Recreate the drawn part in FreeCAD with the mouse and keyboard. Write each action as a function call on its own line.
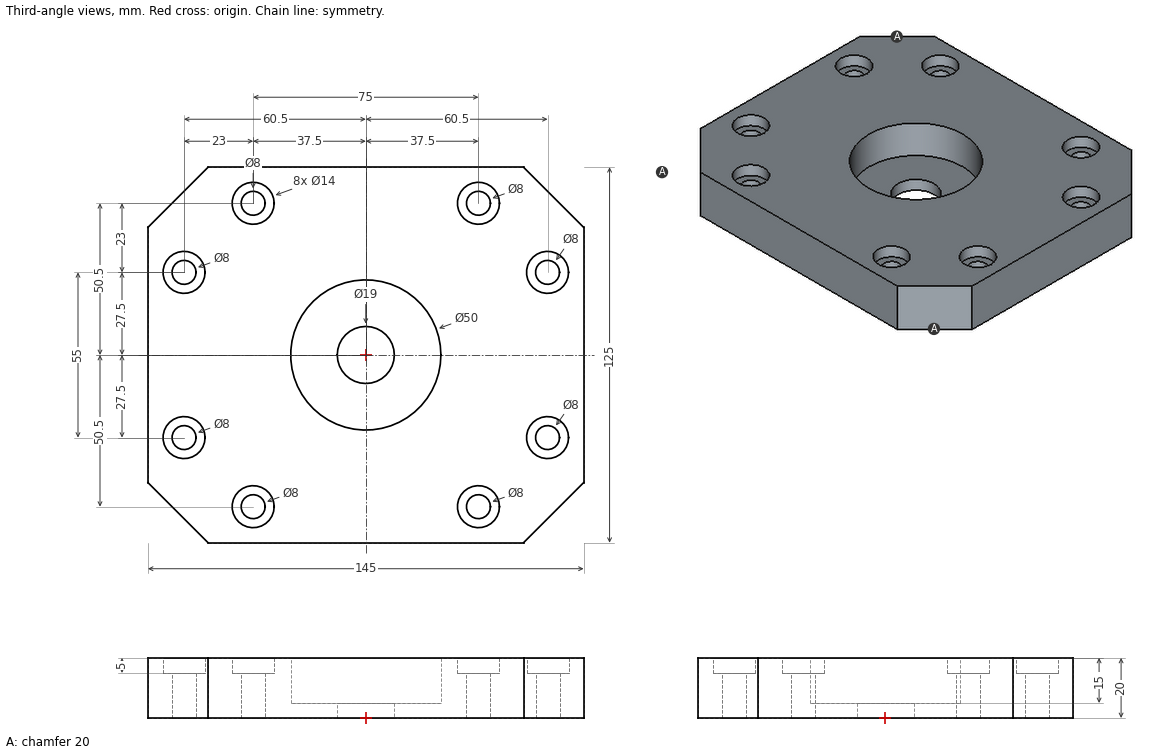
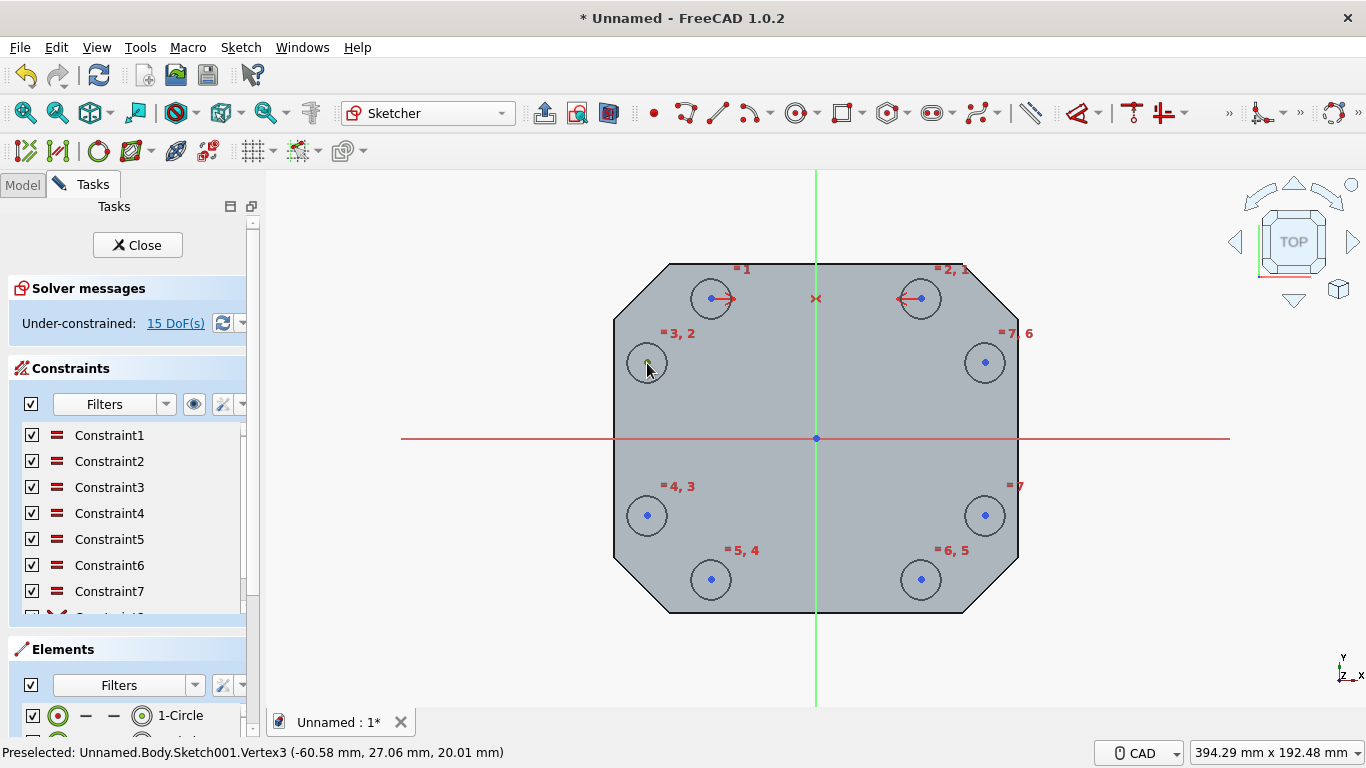
click(647, 516)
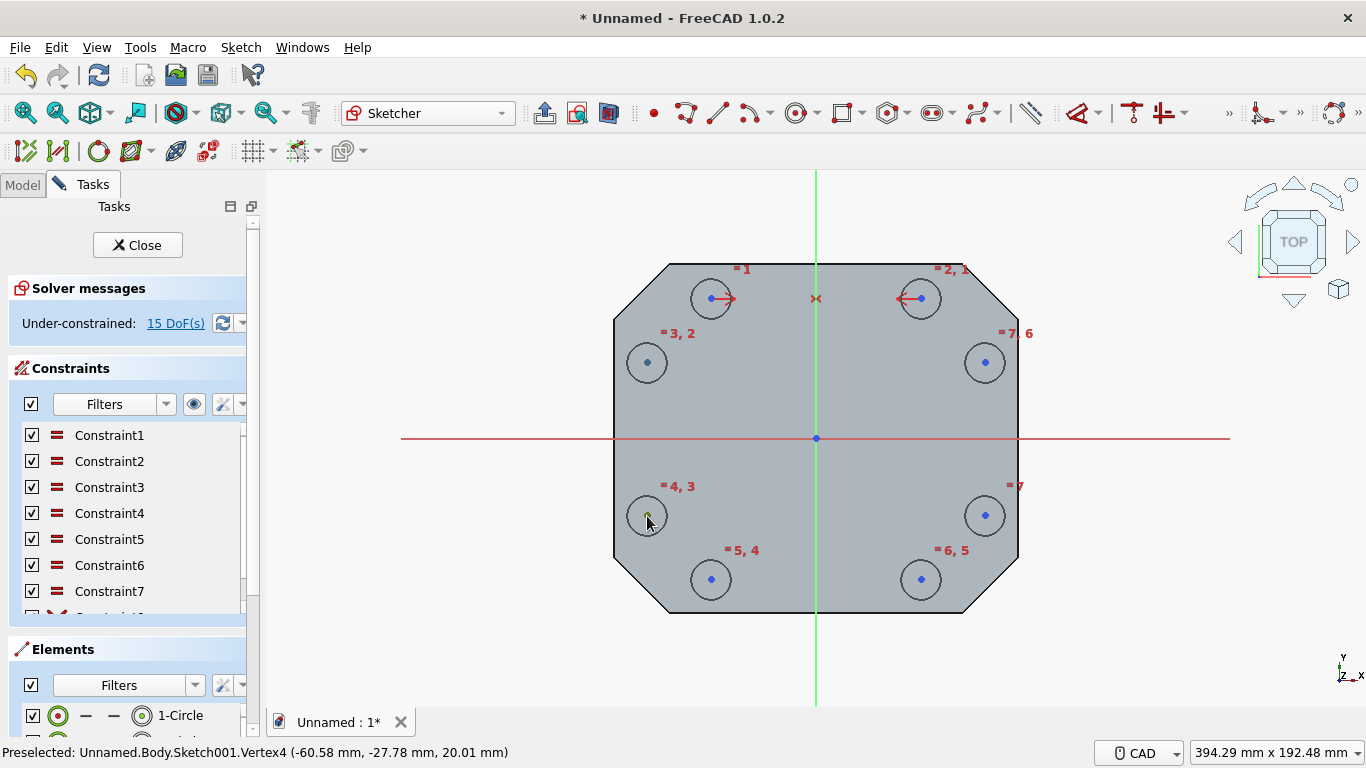
click(424, 438)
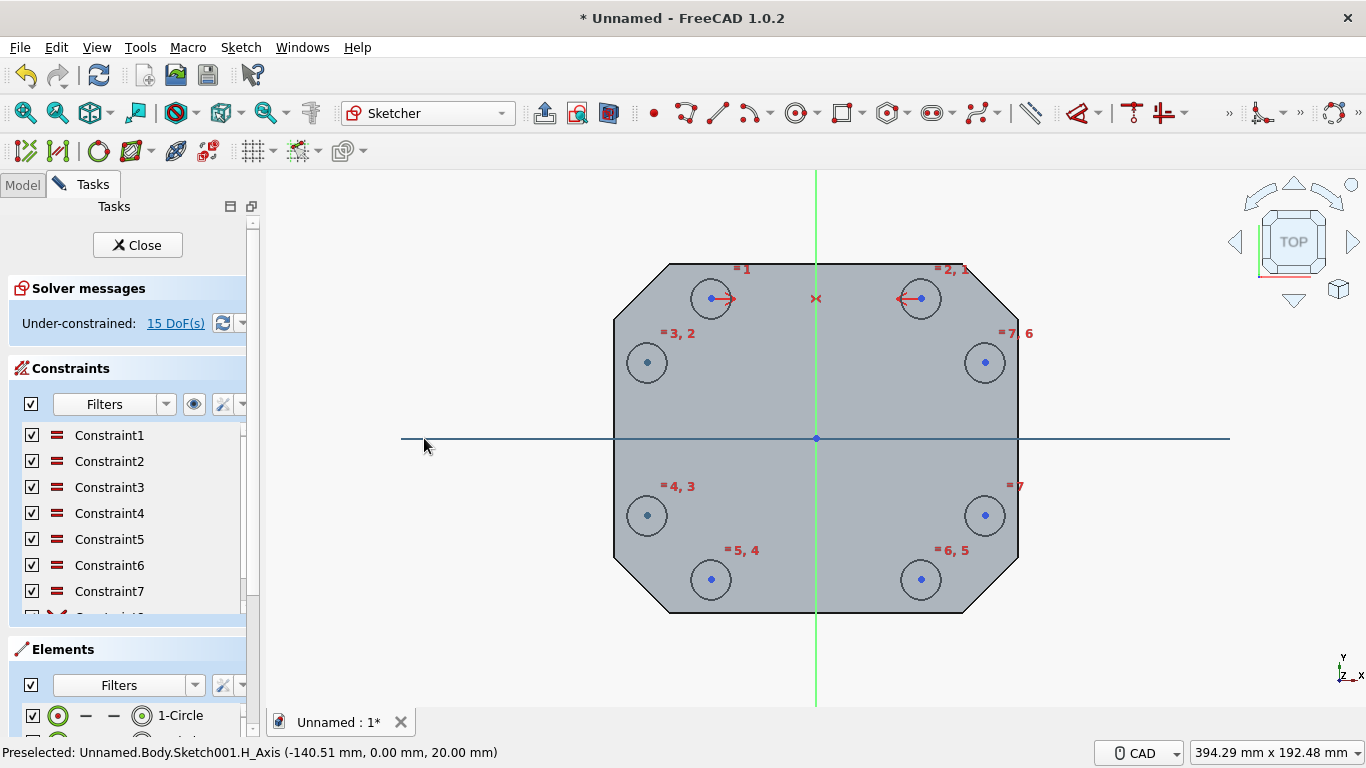
key(s)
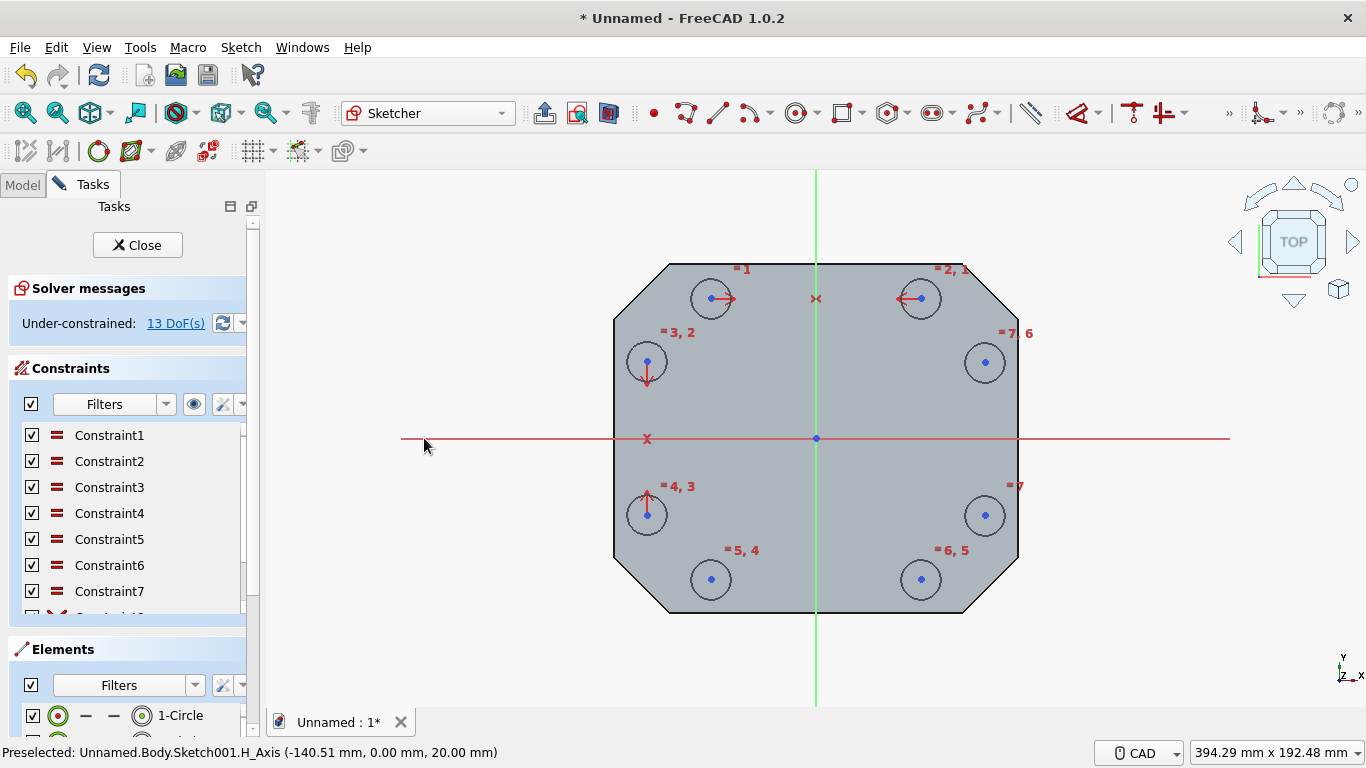
click(711, 299)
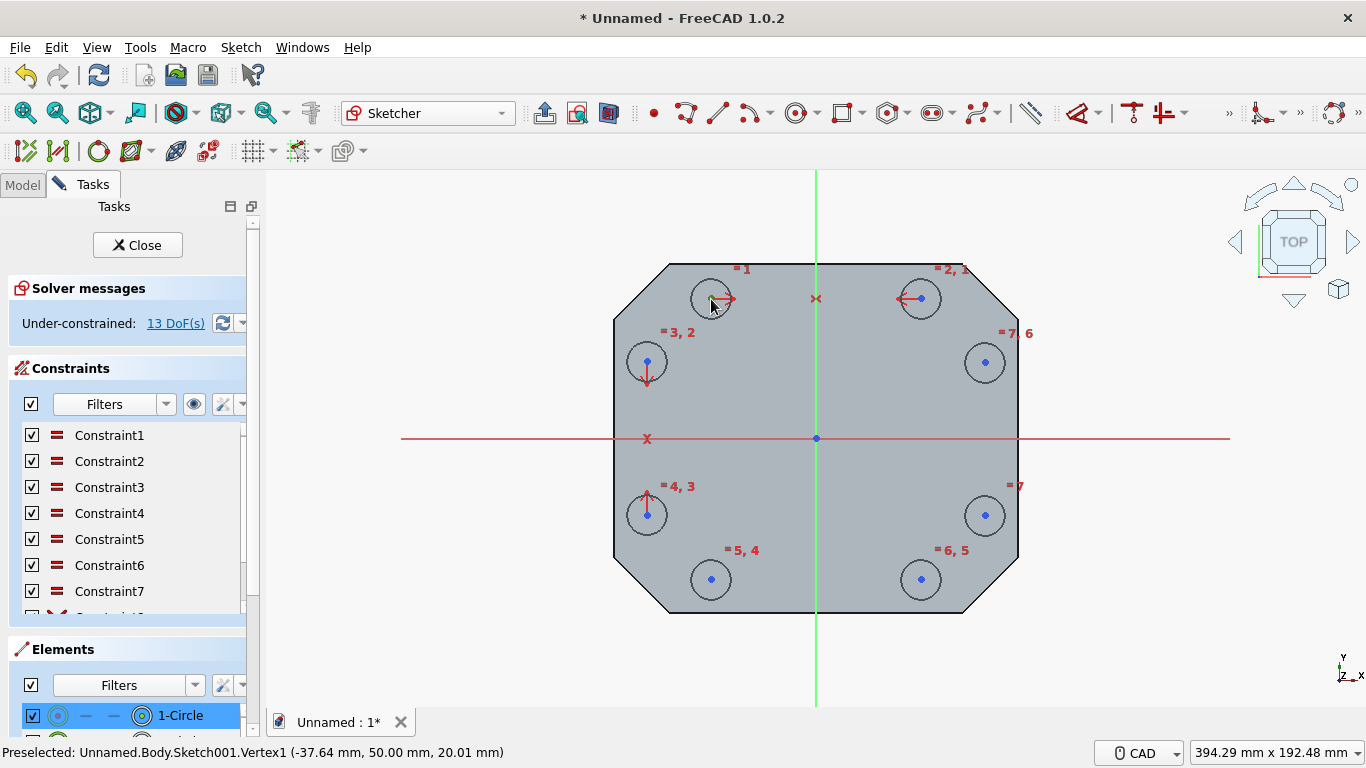
click(711, 580)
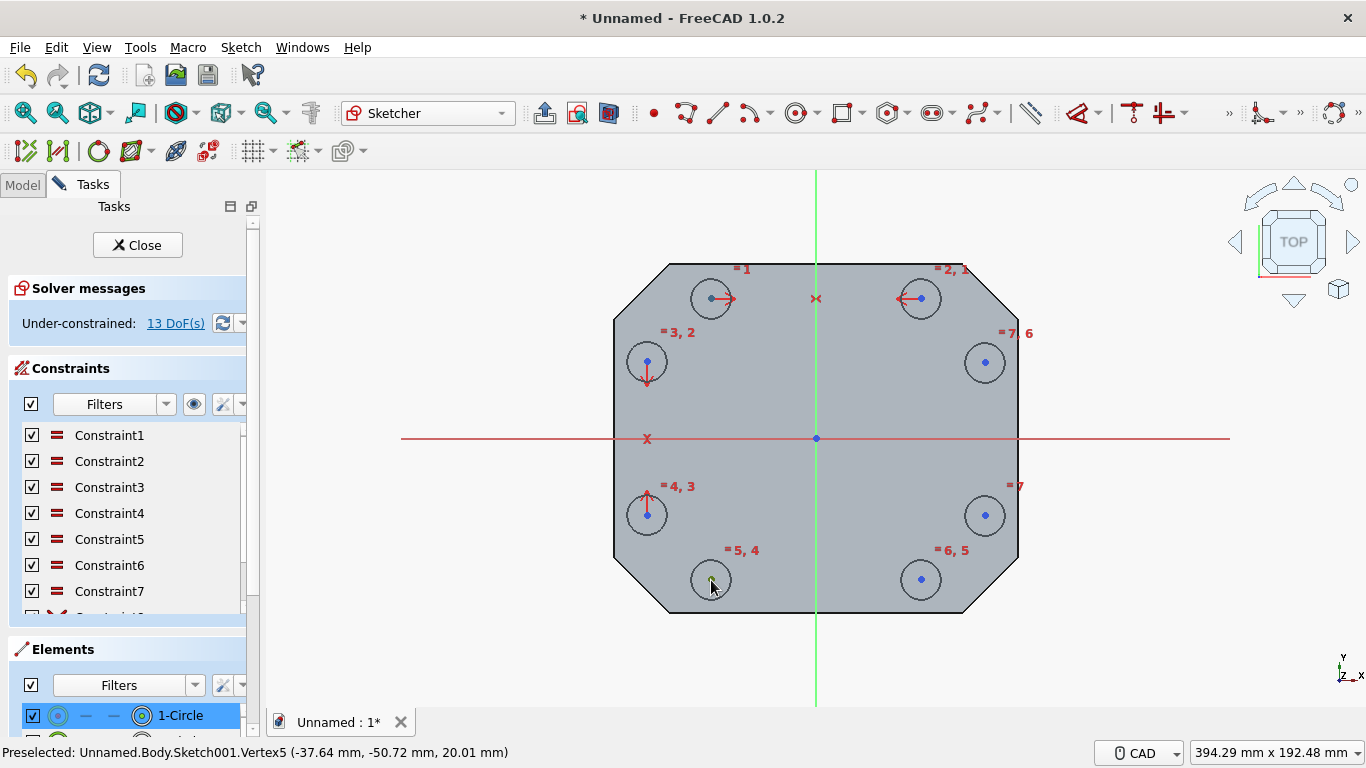
click(424, 438)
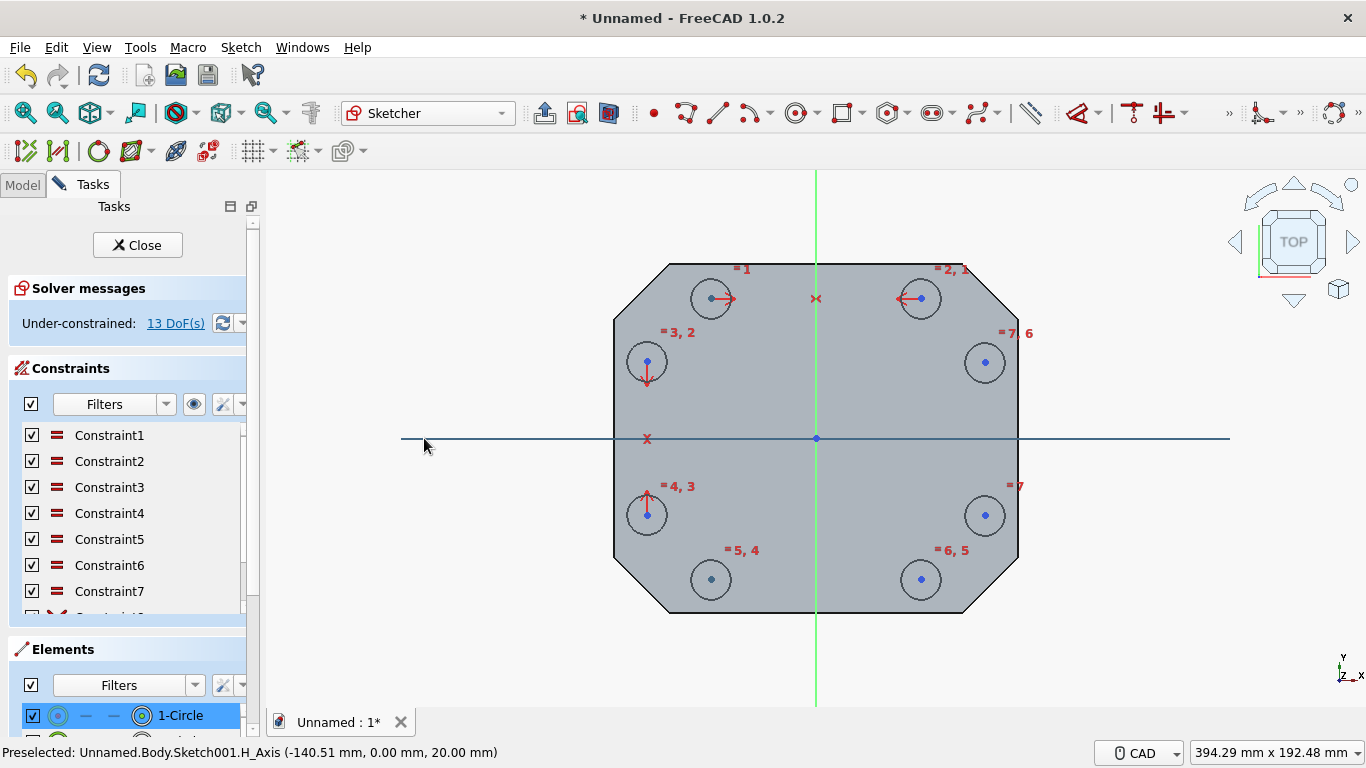
key(s)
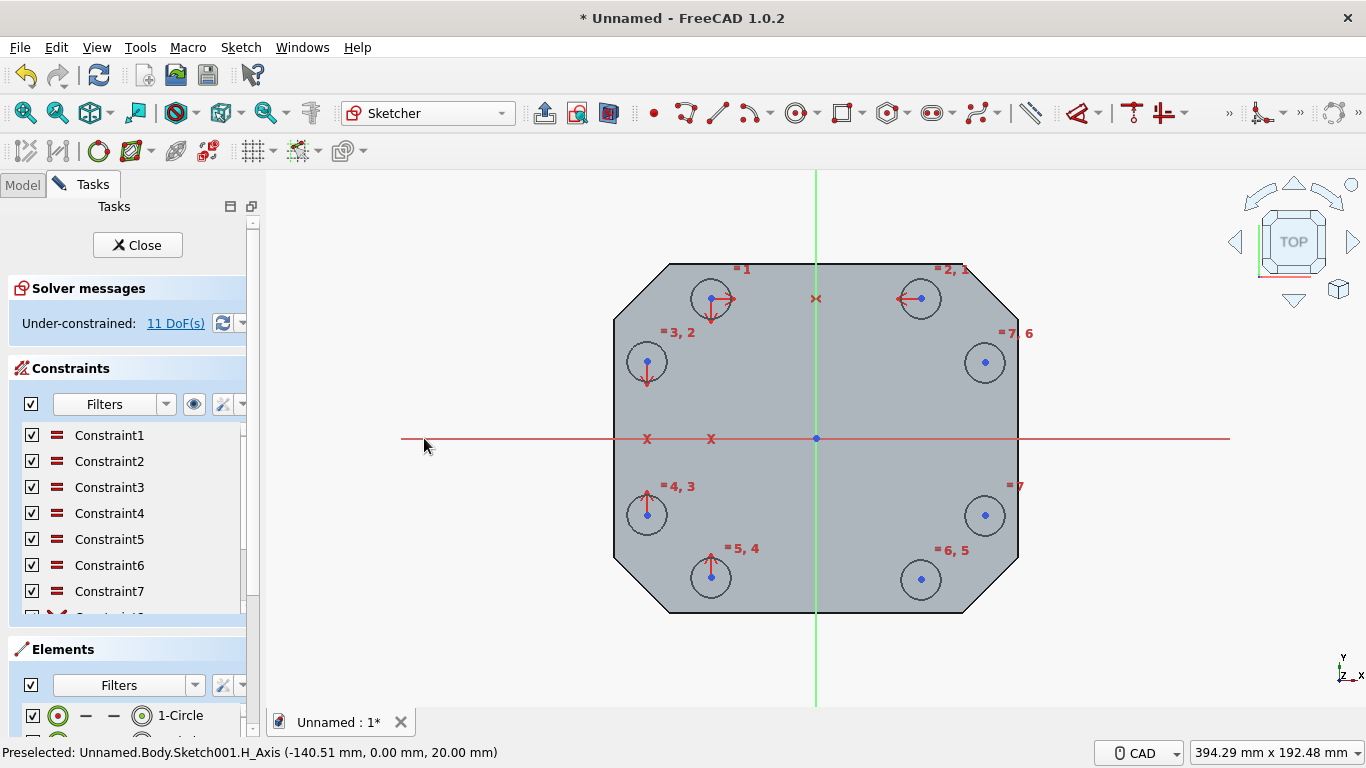
click(921, 299)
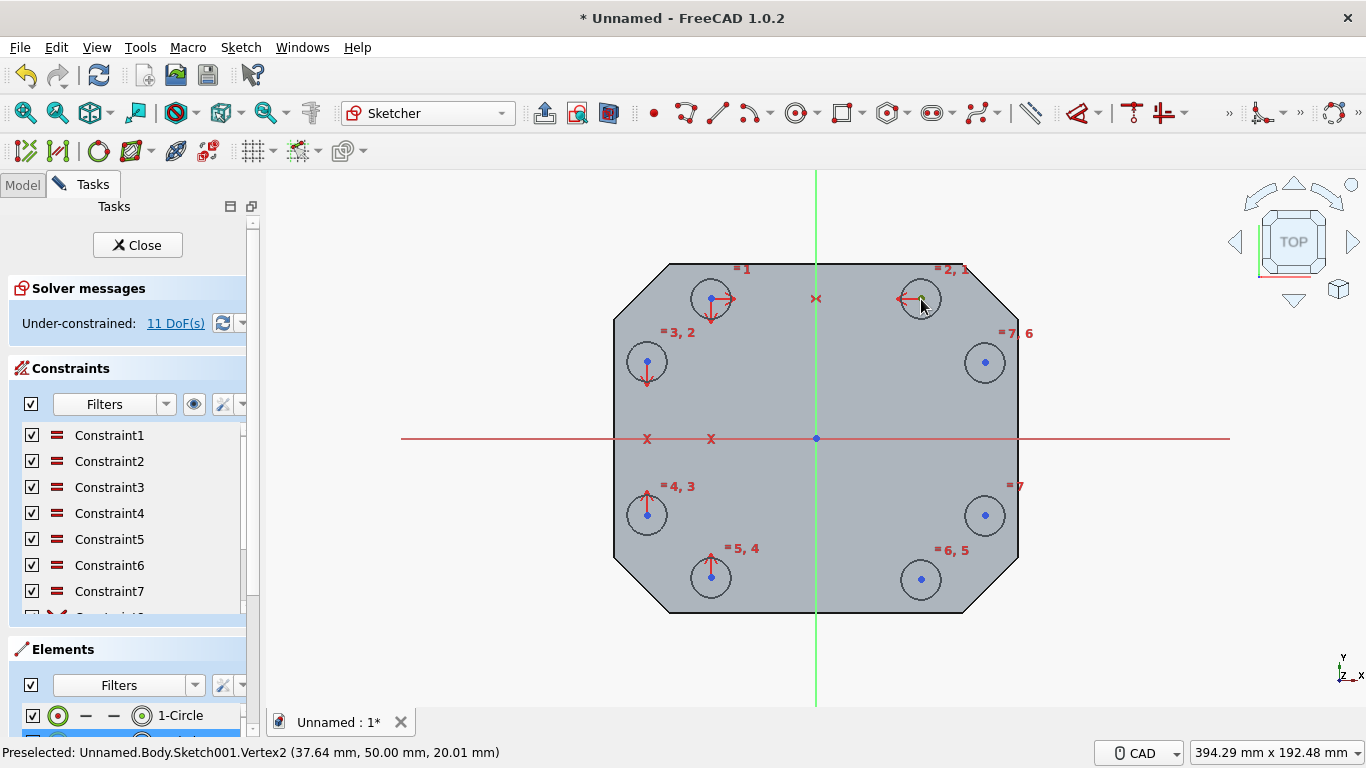
click(921, 580)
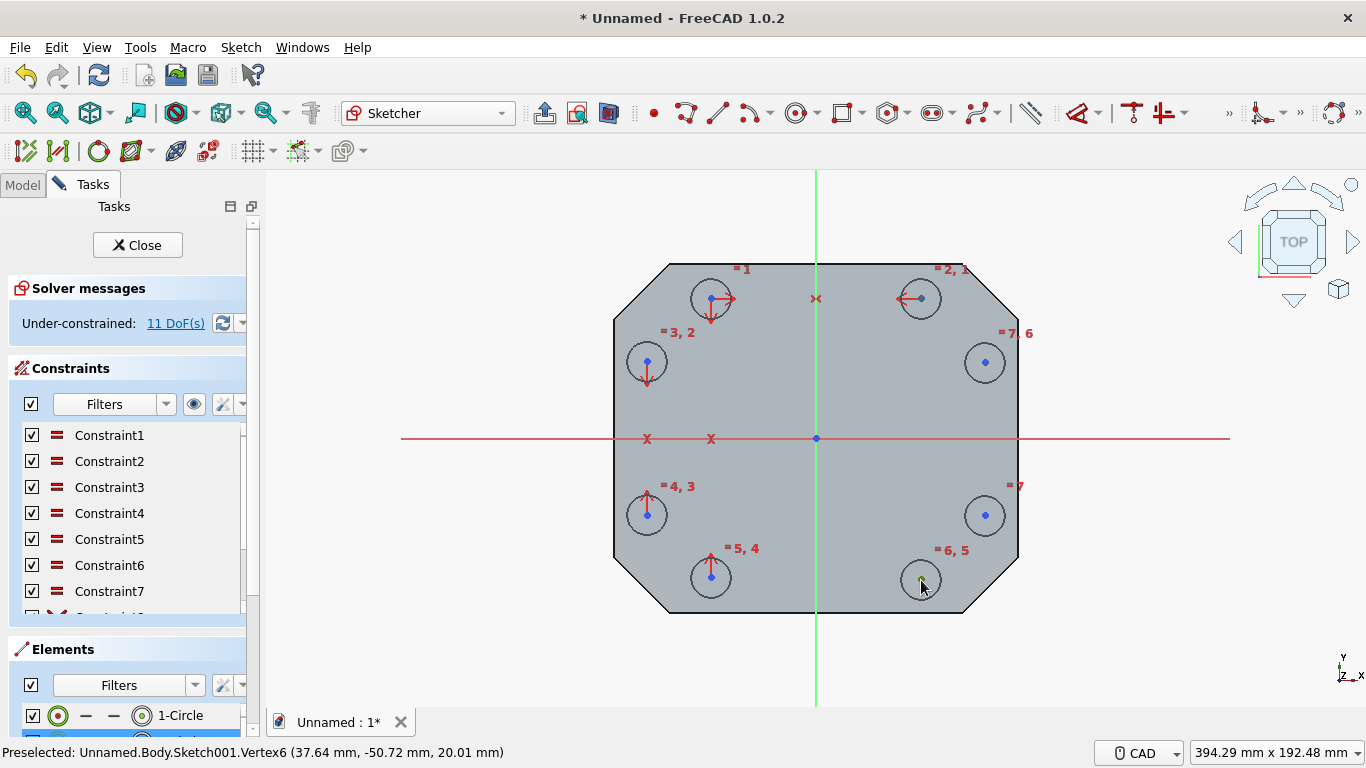
click(424, 438)